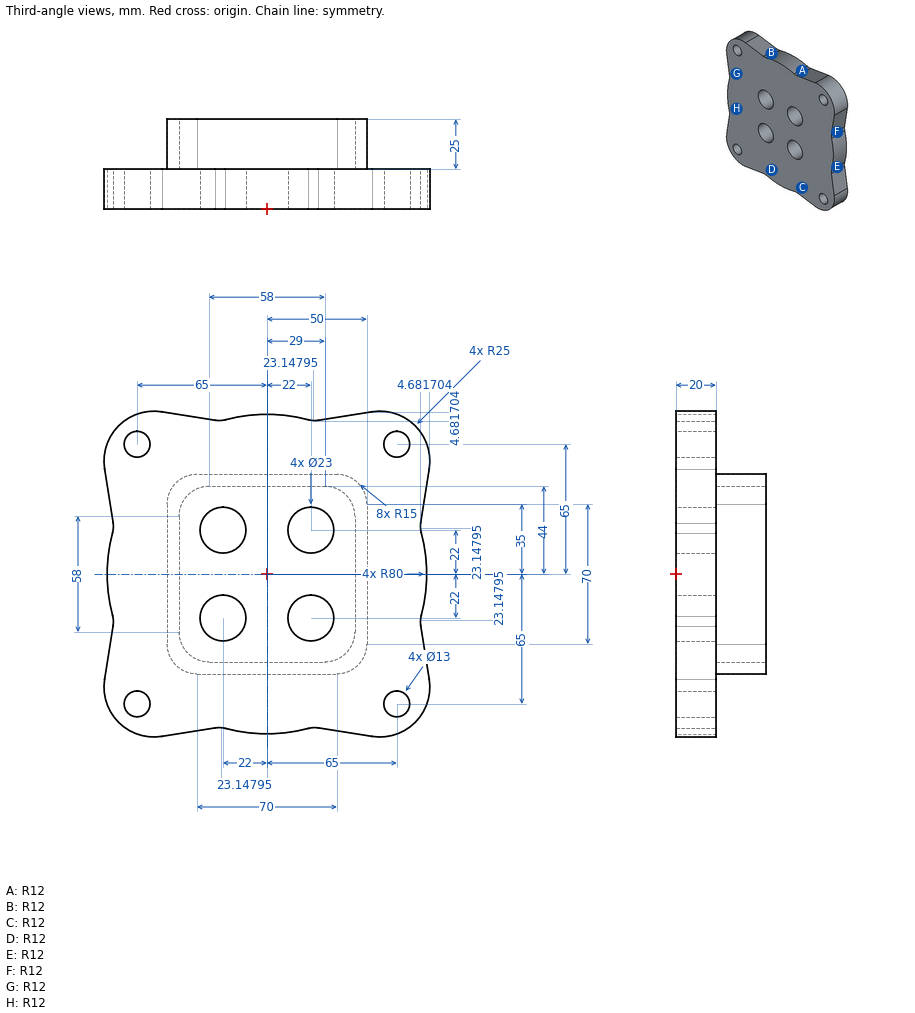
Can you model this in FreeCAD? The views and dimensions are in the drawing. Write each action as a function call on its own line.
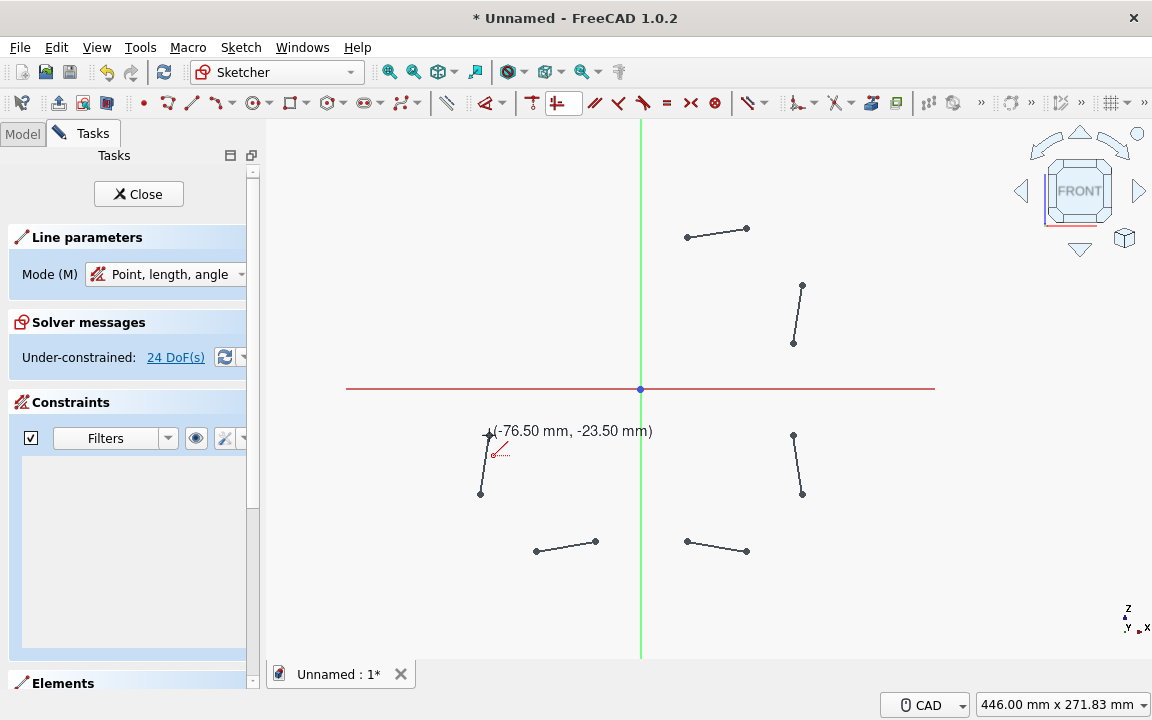
click(489, 343)
click(480, 285)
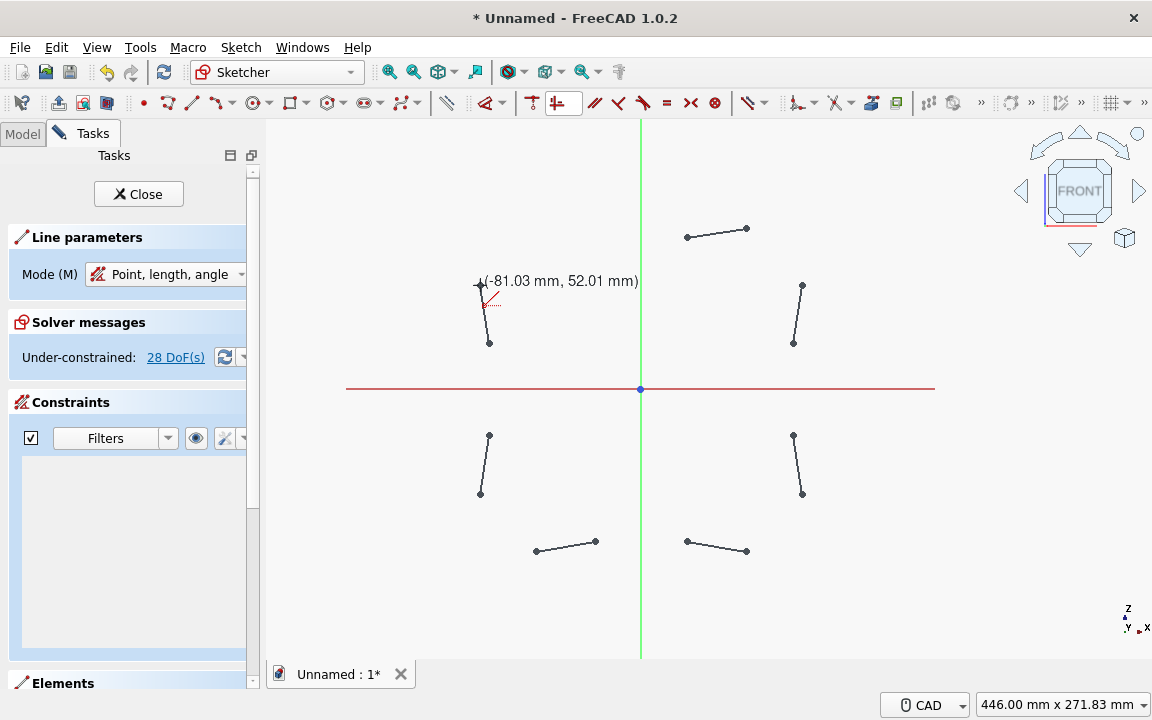
click(536, 228)
click(595, 237)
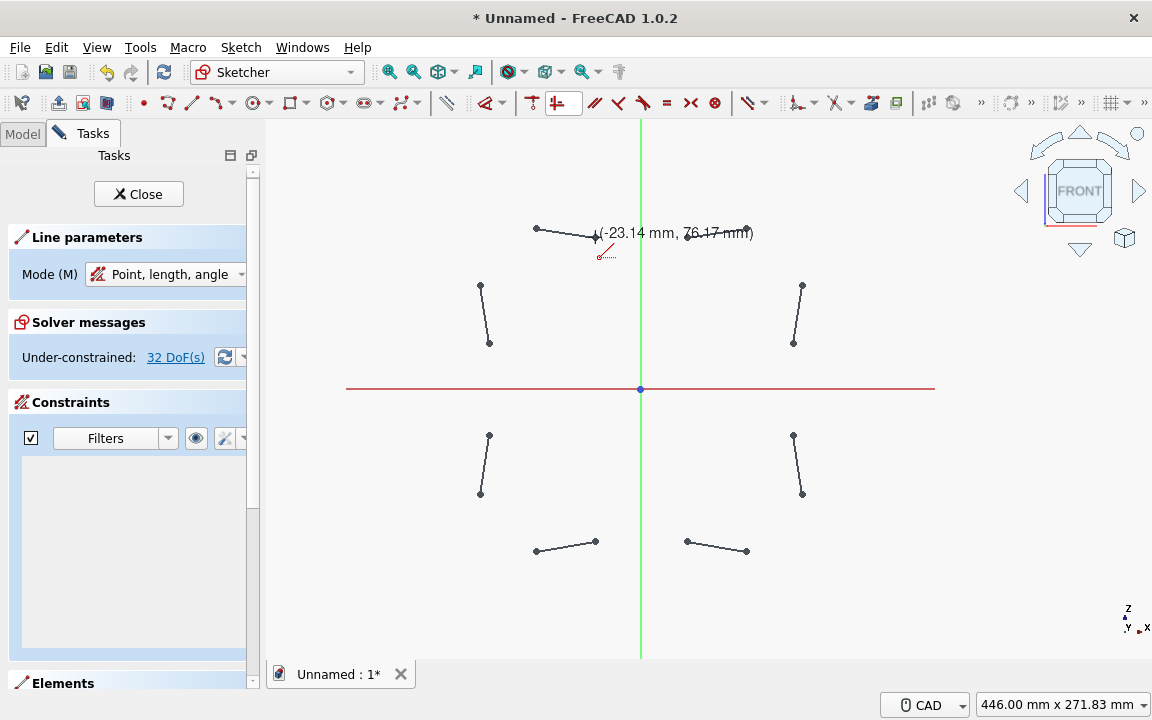
click(216, 104)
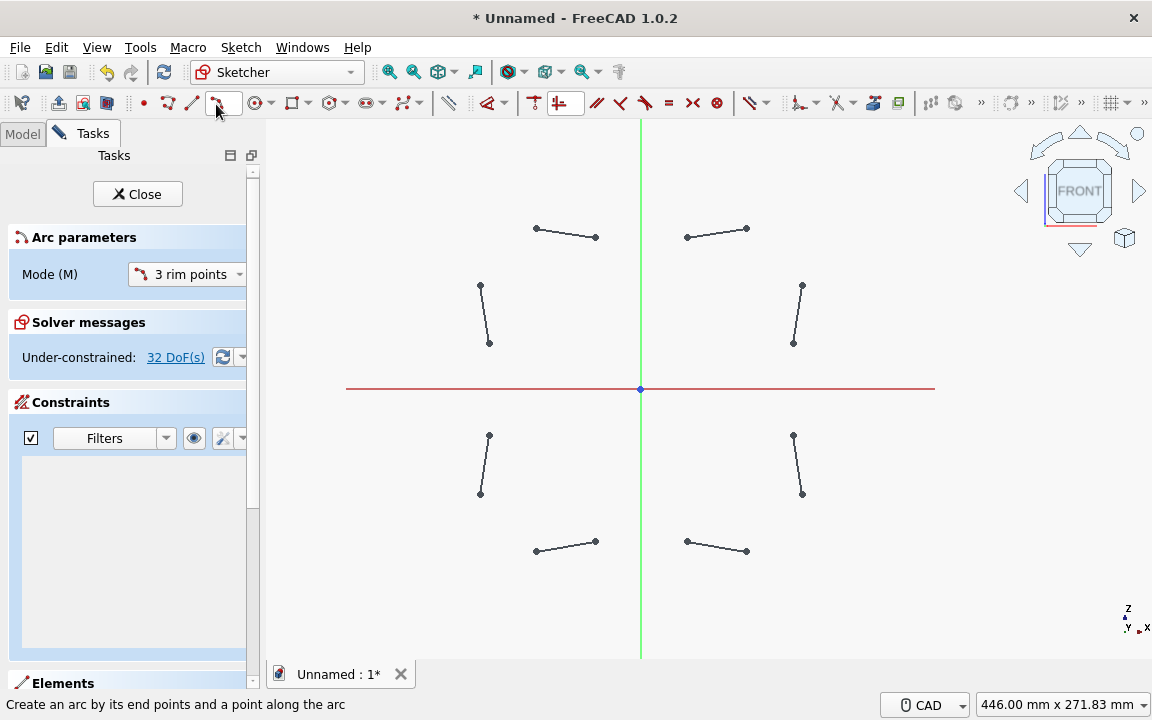
click(746, 229)
click(802, 286)
click(788, 242)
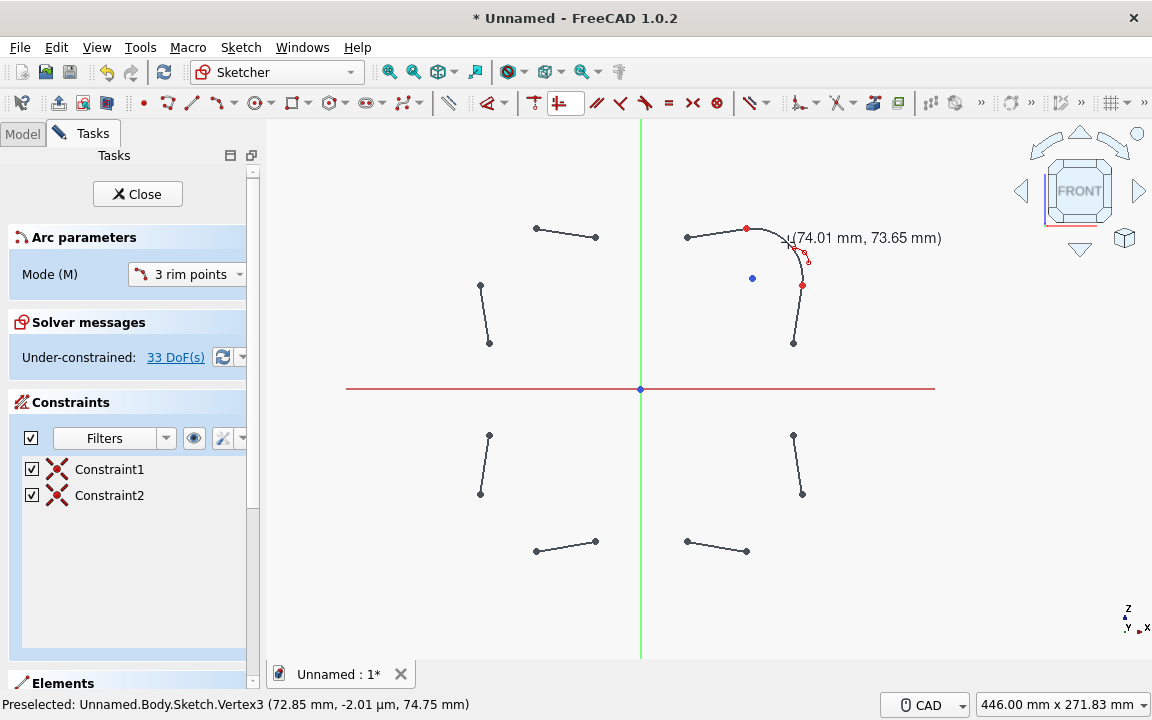
click(793, 344)
click(793, 436)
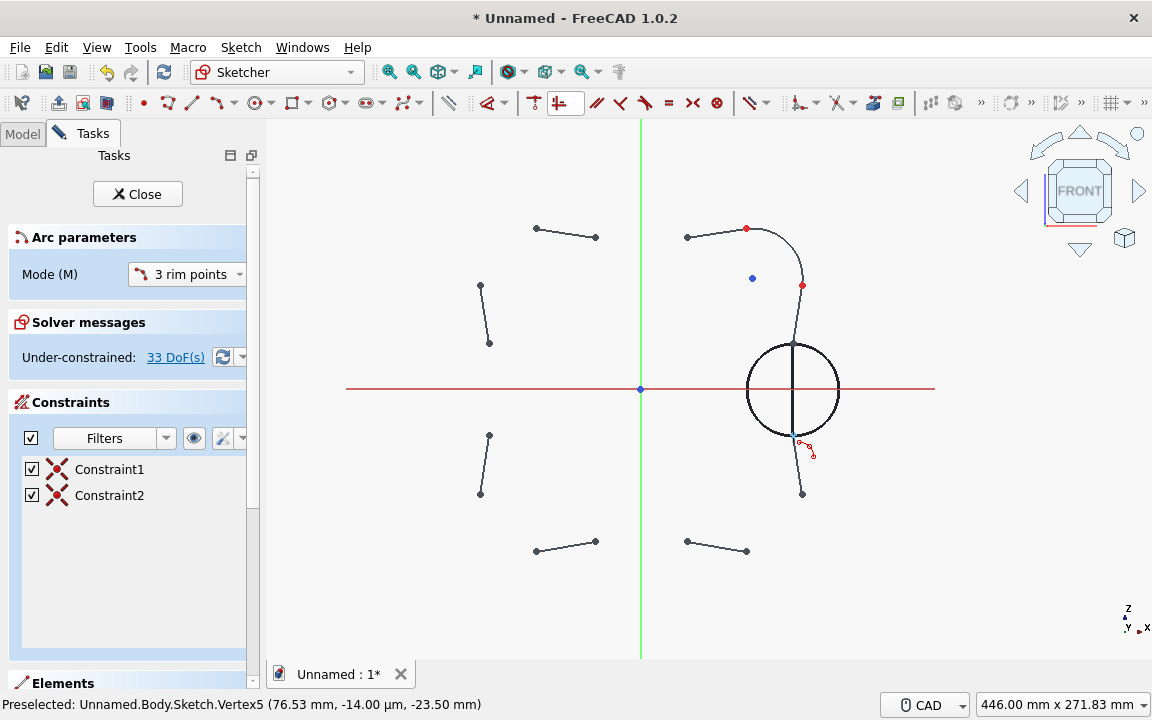
scroll(800, 399, up, 5)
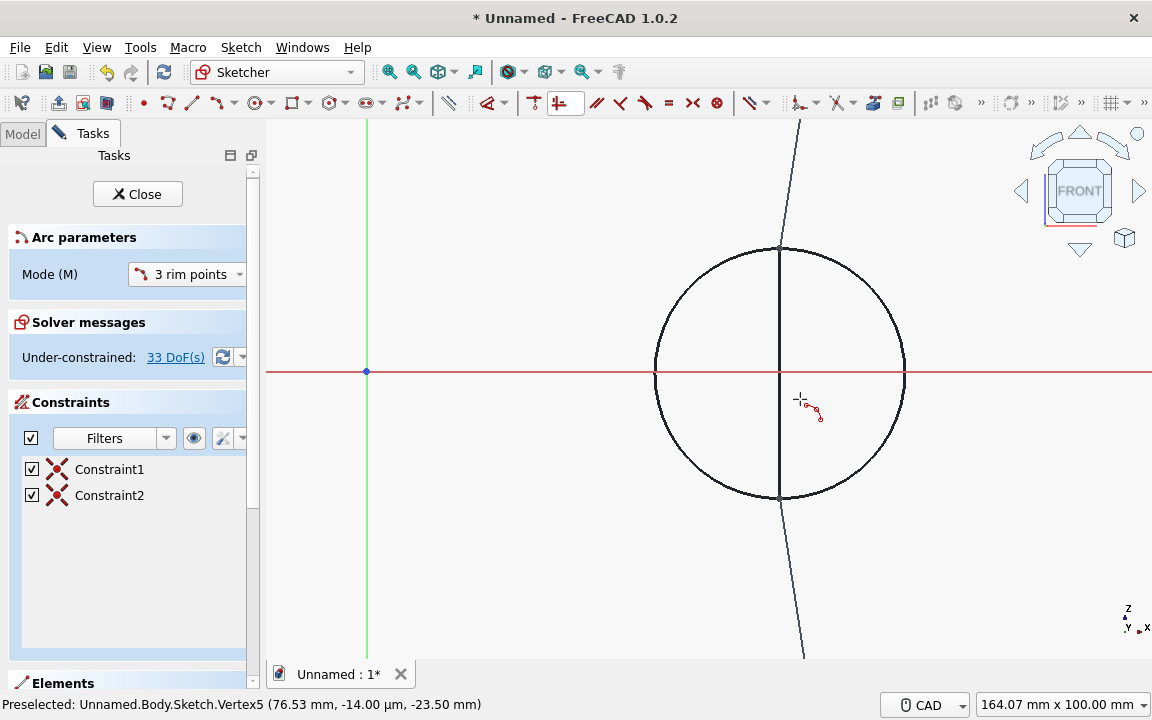
click(798, 397)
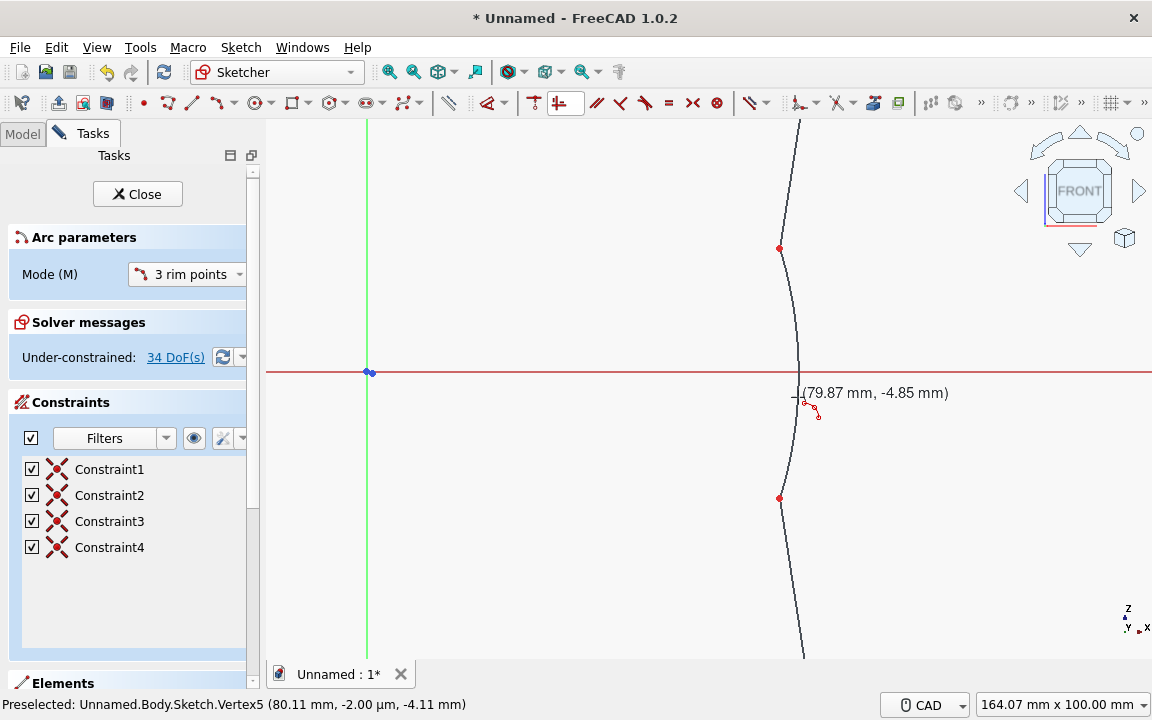
scroll(800, 399, down, 5)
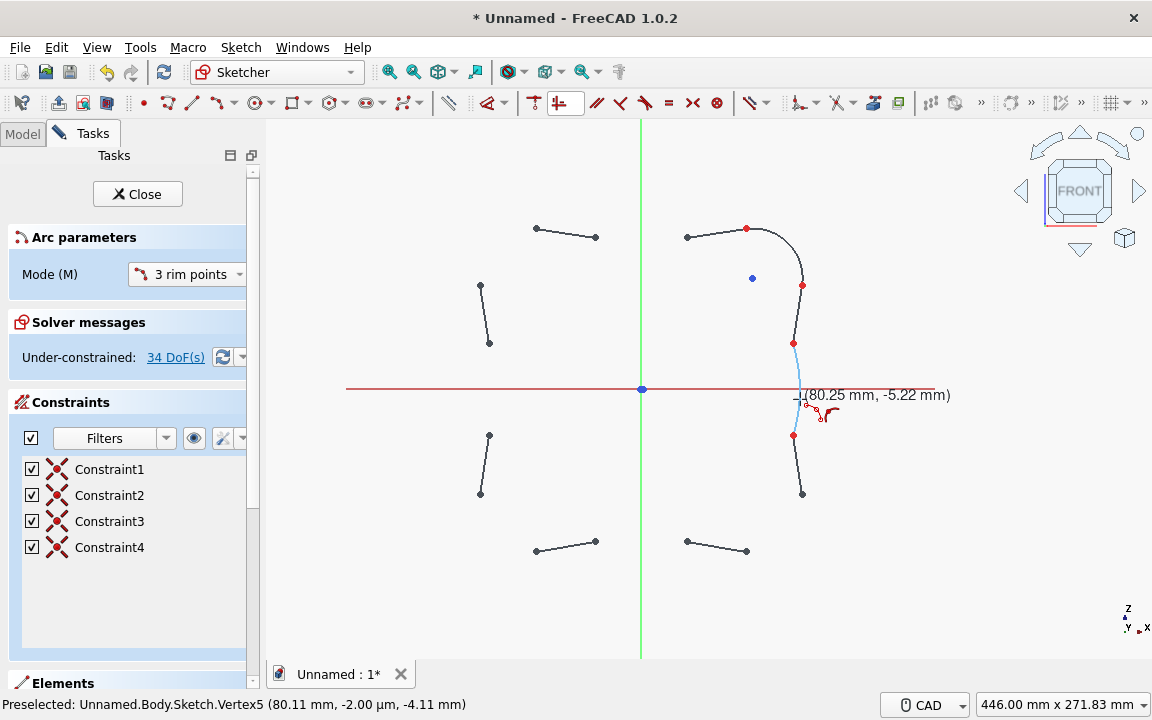
click(802, 495)
click(746, 552)
click(788, 537)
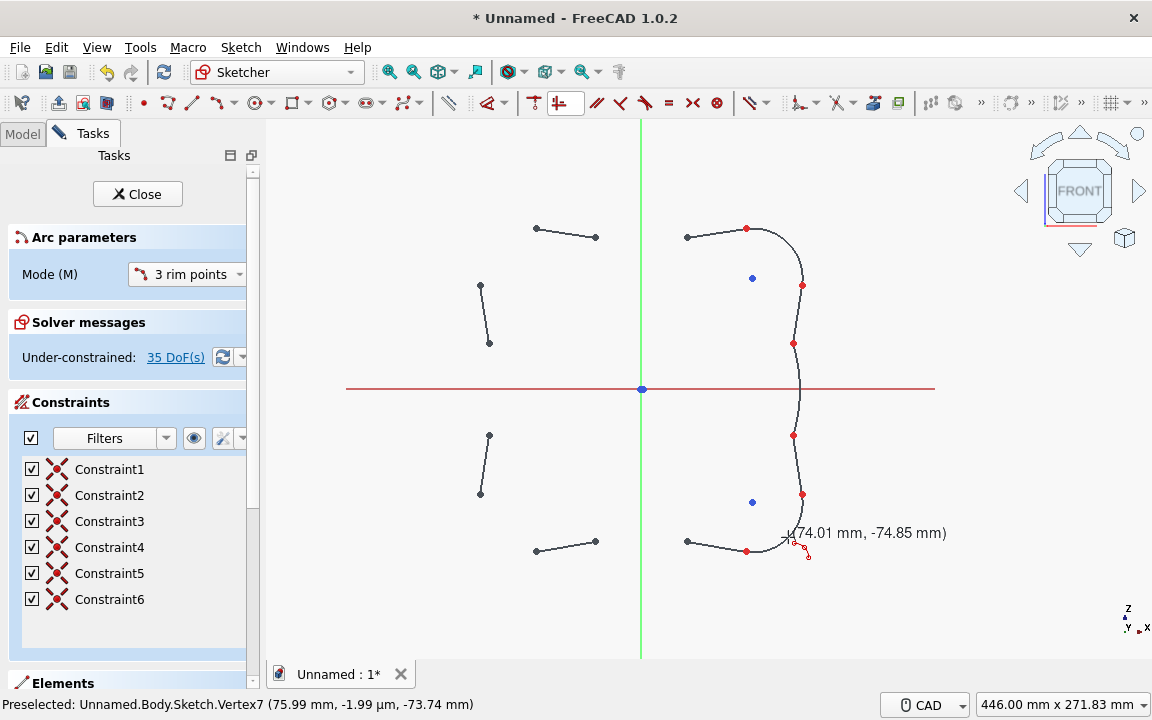
click(687, 542)
click(595, 542)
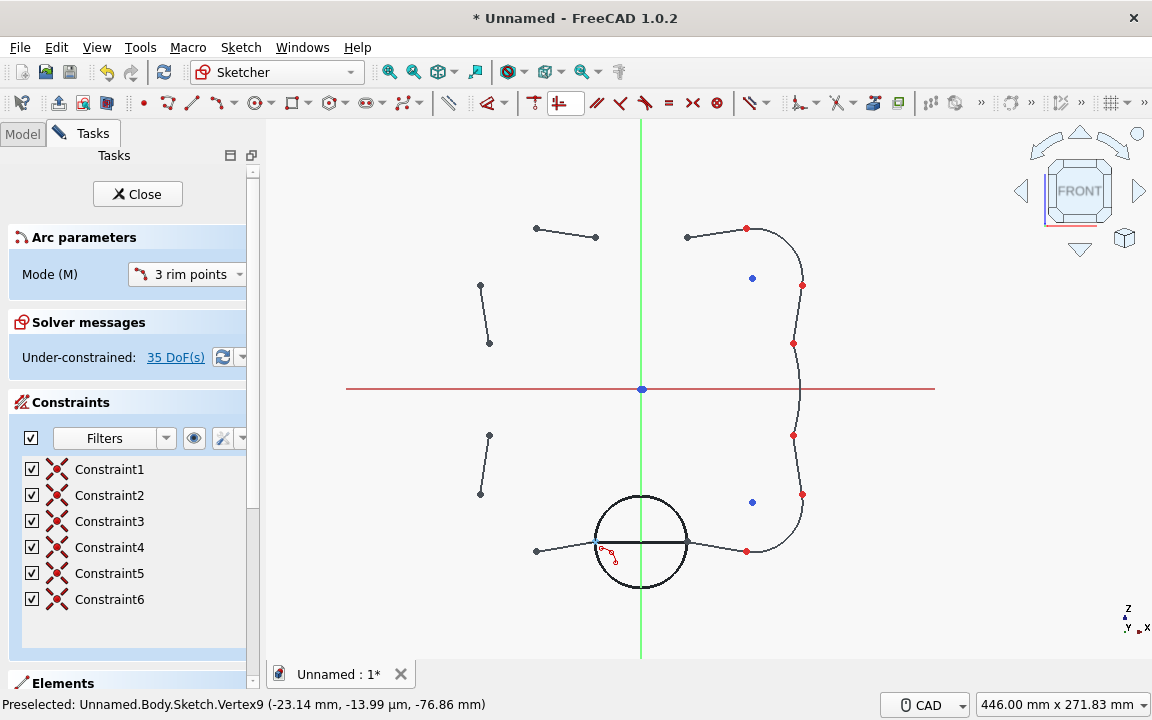
scroll(632, 548, up, 5)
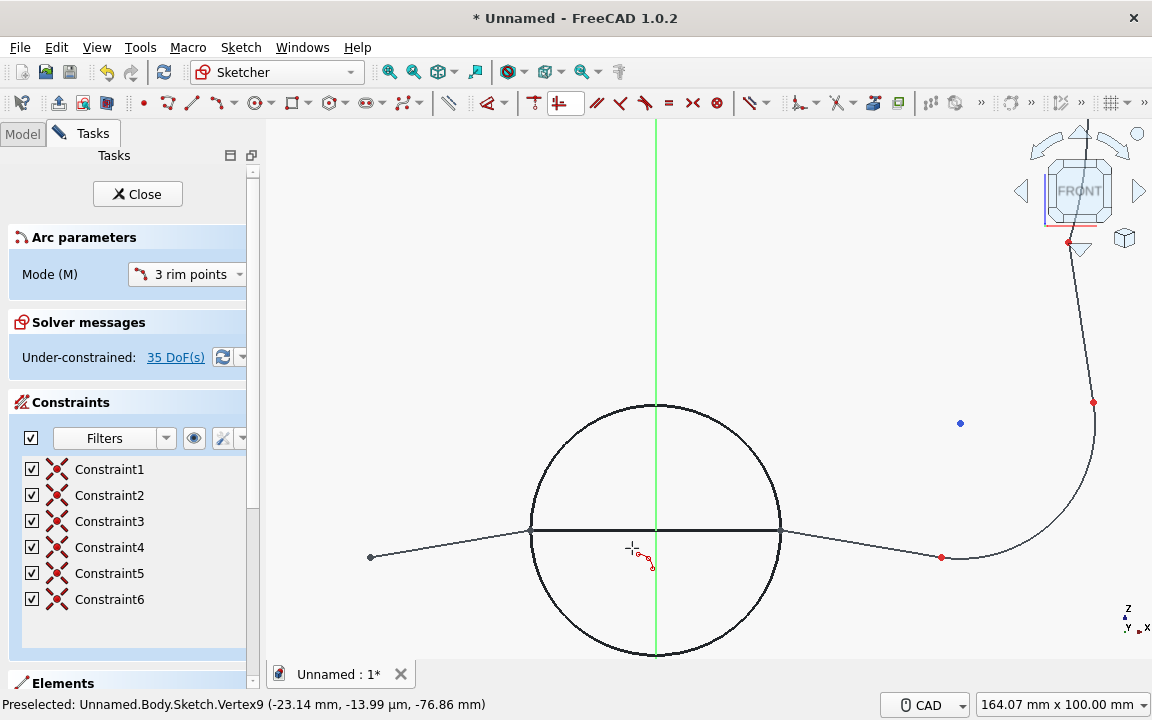
click(630, 547)